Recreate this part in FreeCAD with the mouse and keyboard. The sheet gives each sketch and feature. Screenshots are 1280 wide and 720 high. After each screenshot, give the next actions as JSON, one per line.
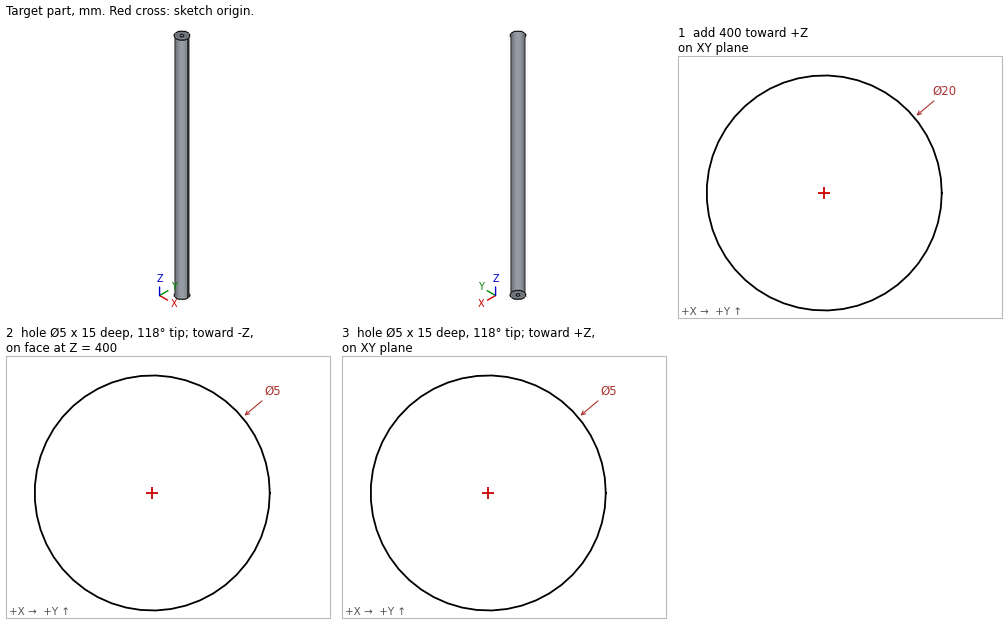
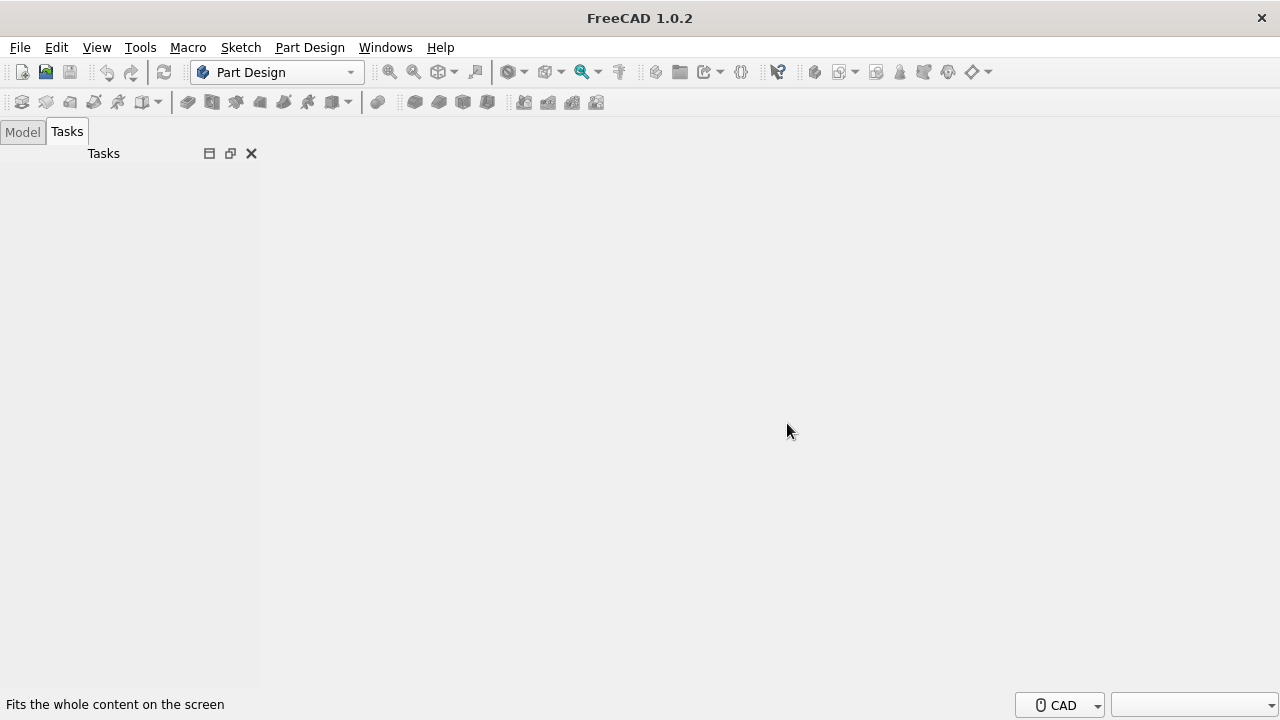
{"action": "key", "text": "ctrl+n"}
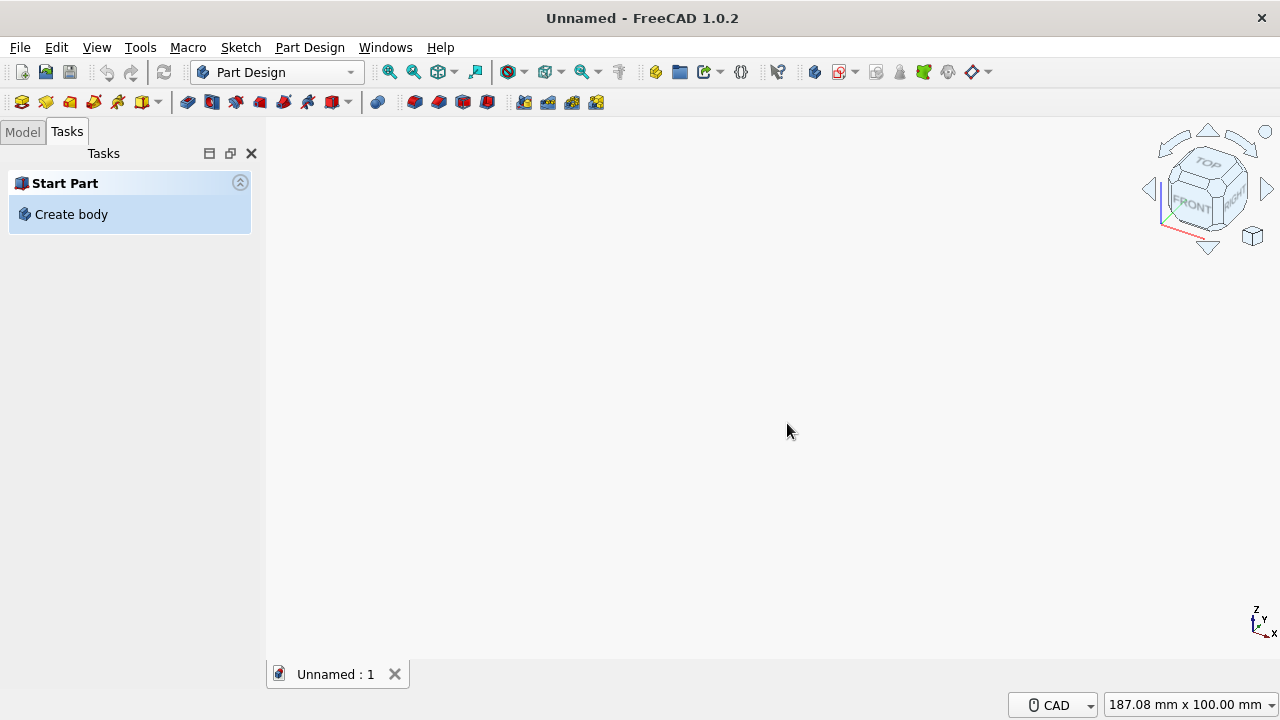
{"action": "left_click", "coordinate": [840, 72]}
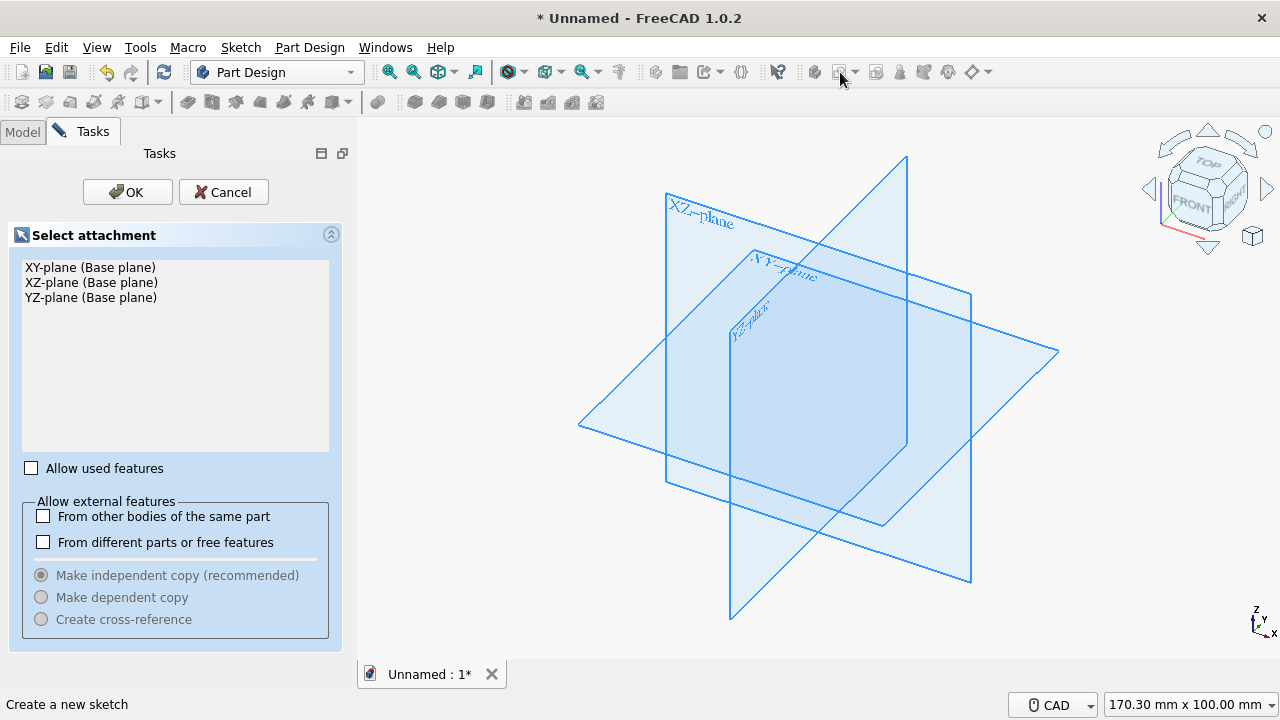
{"action": "left_click", "coordinate": [82, 268]}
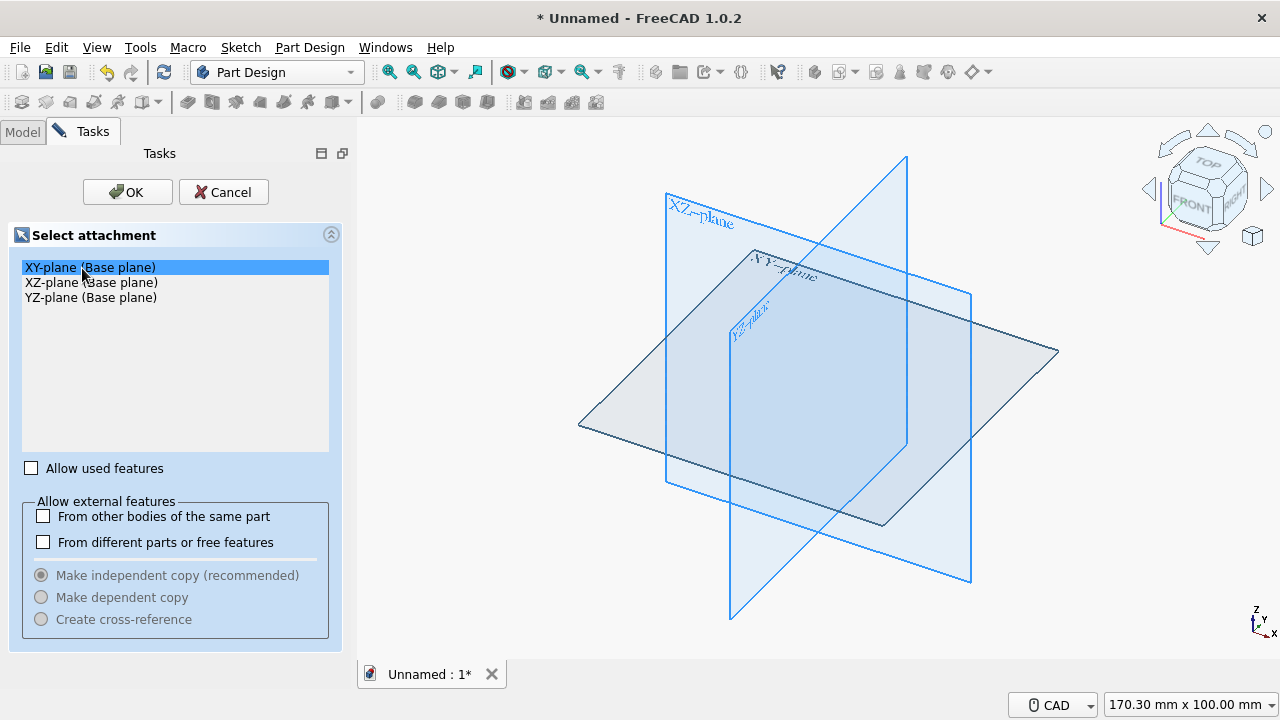
{"action": "left_click", "coordinate": [128, 192]}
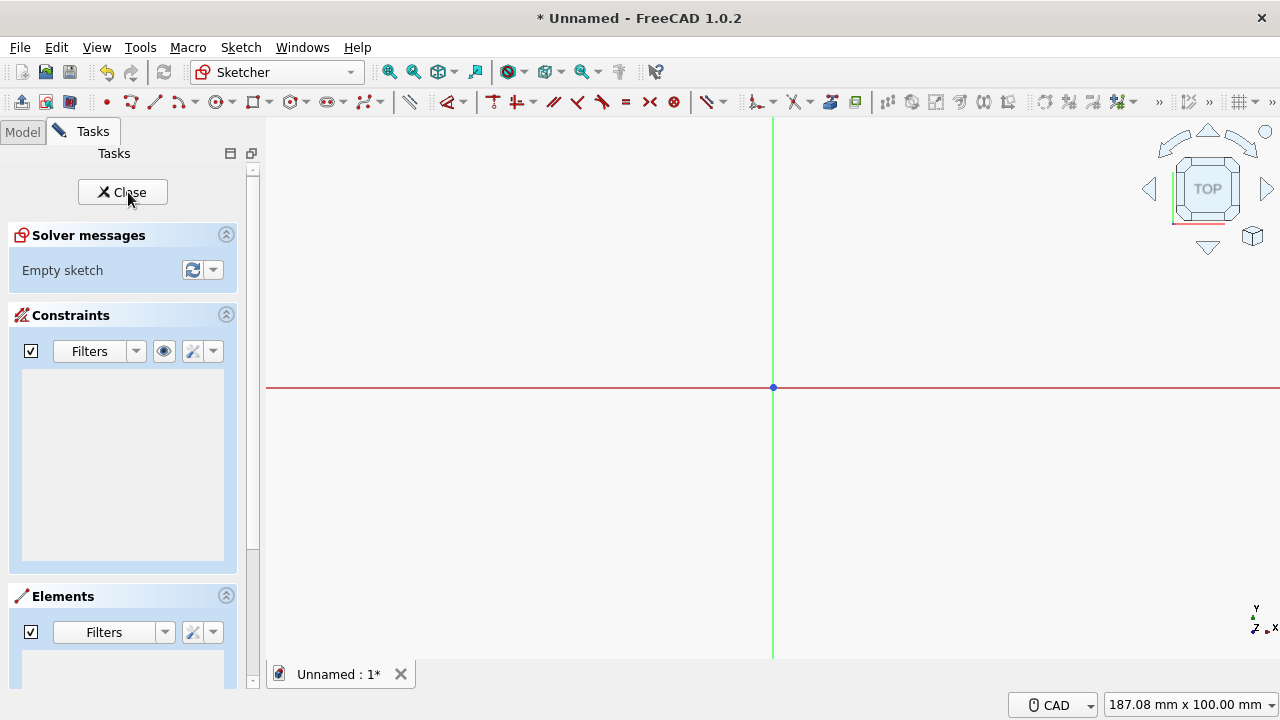
{"action": "scroll", "coordinate": [803, 388], "scroll_direction": "up", "scroll_amount": 6}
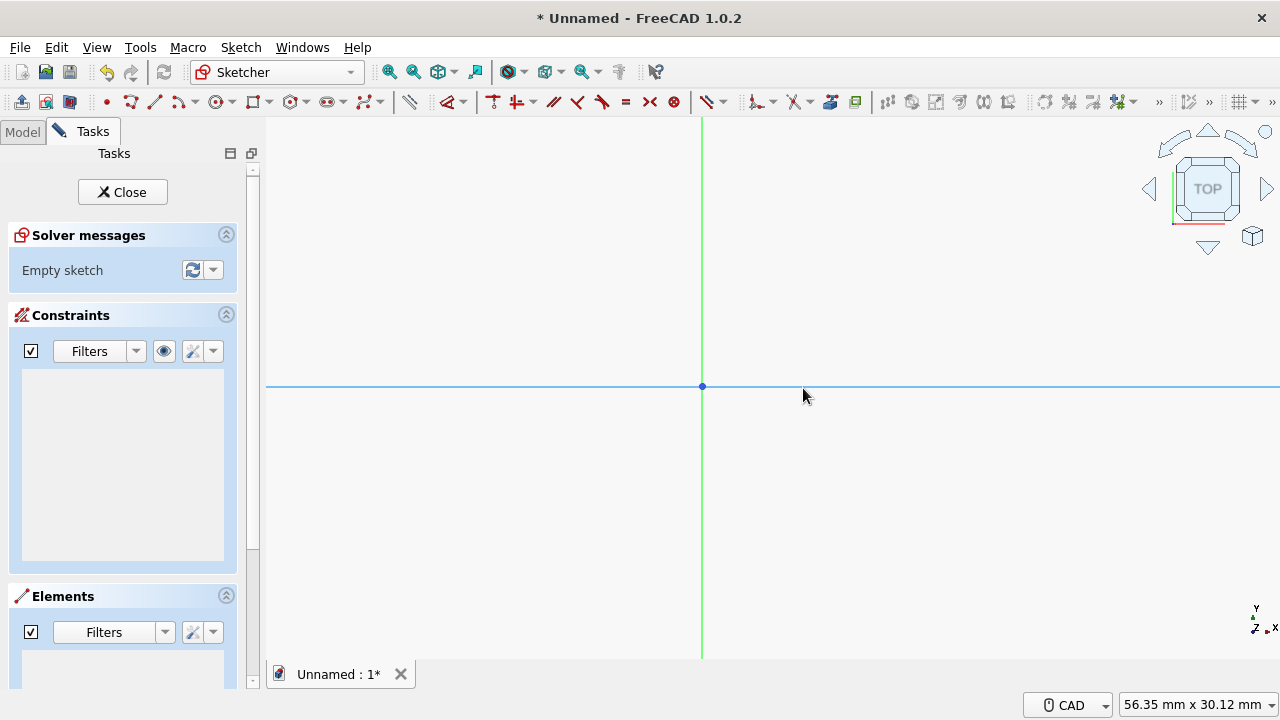
{"action": "left_click", "coordinate": [216, 102]}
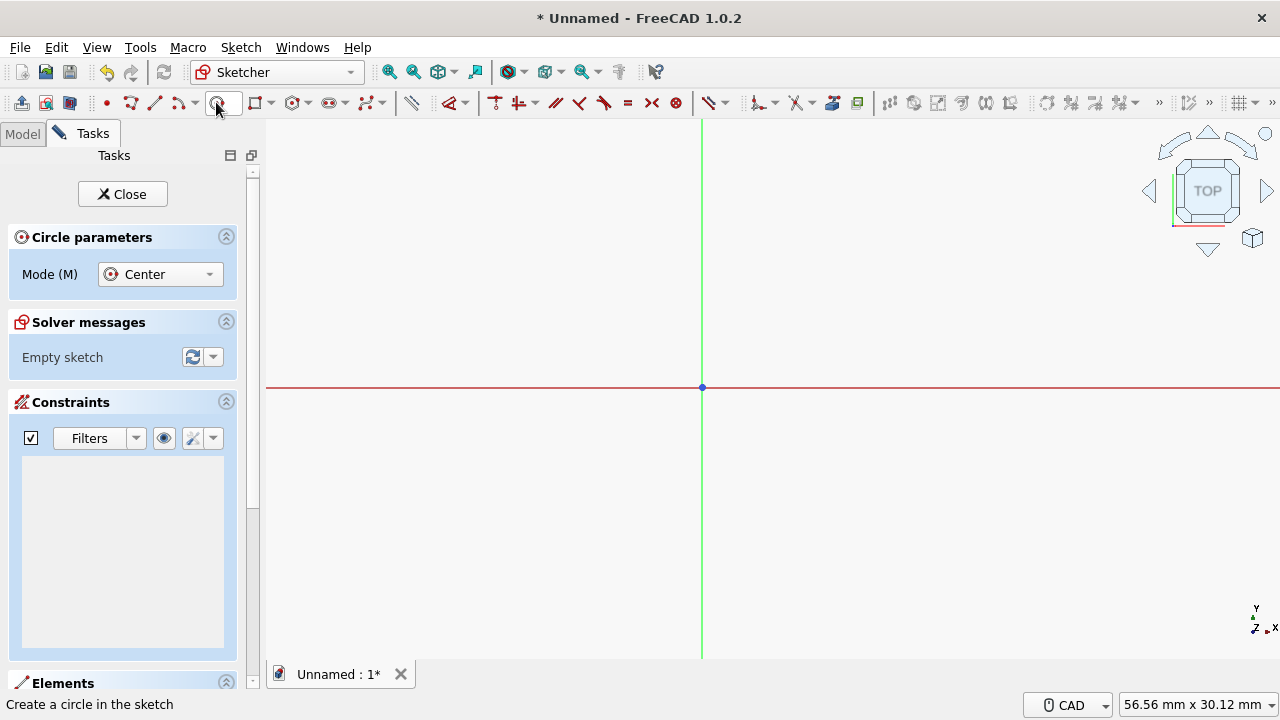
{"action": "left_click", "coordinate": [702, 388]}
{"action": "mouse_move", "coordinate": [829, 261]}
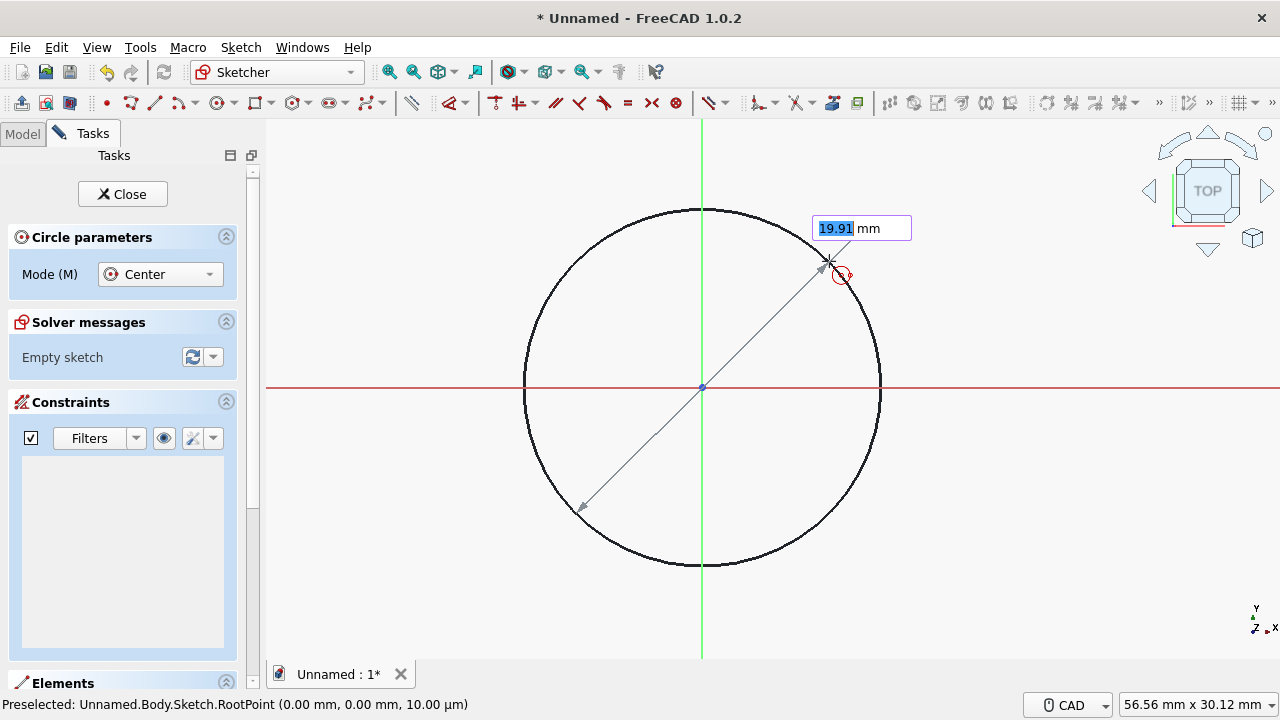
{"action": "type", "text": "20"}
{"action": "key", "text": "Return"}
{"action": "key", "text": "Escape"}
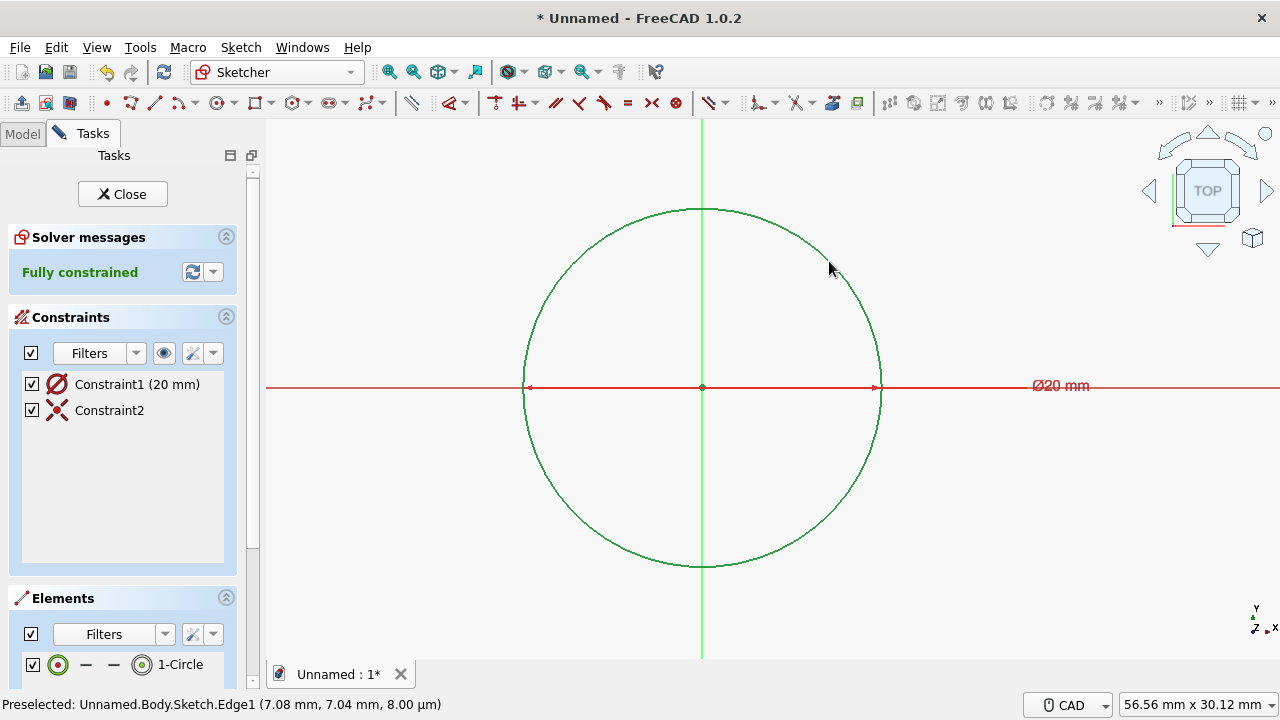
{"action": "left_click", "coordinate": [123, 194]}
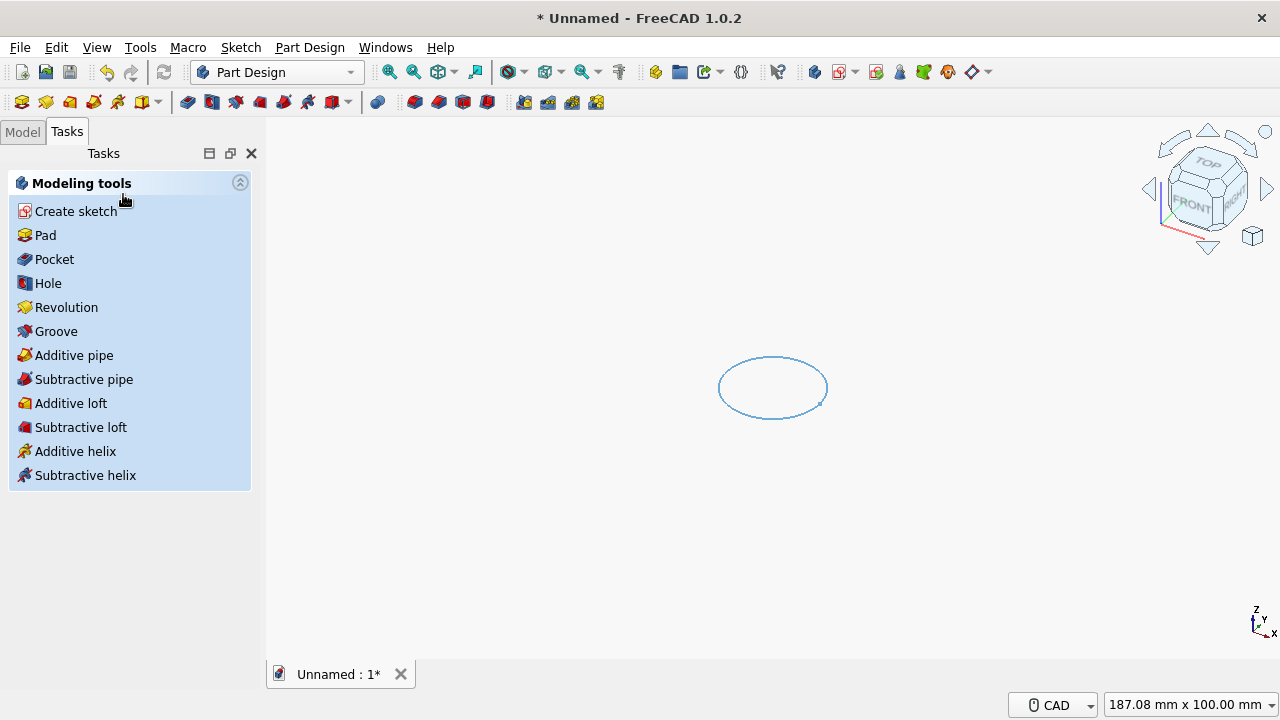
{"action": "left_click", "coordinate": [22, 102]}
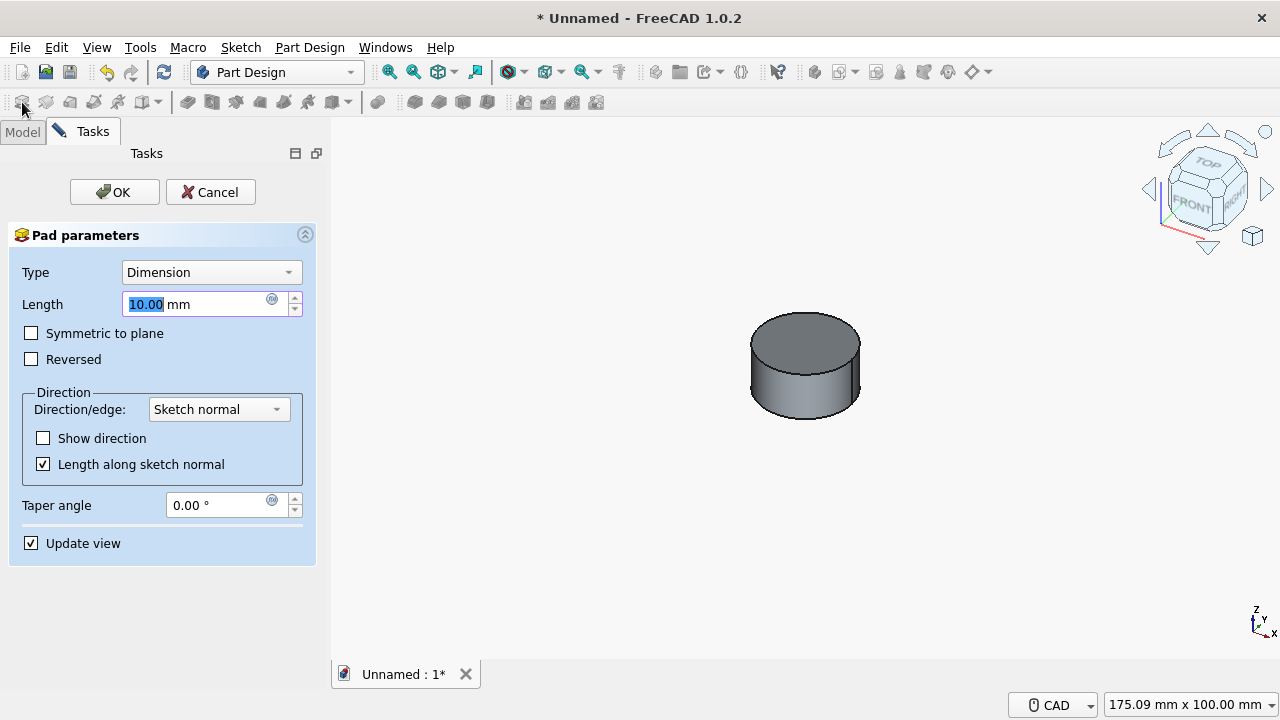
{"action": "type", "text": "400"}
{"action": "key", "text": "Tab"}